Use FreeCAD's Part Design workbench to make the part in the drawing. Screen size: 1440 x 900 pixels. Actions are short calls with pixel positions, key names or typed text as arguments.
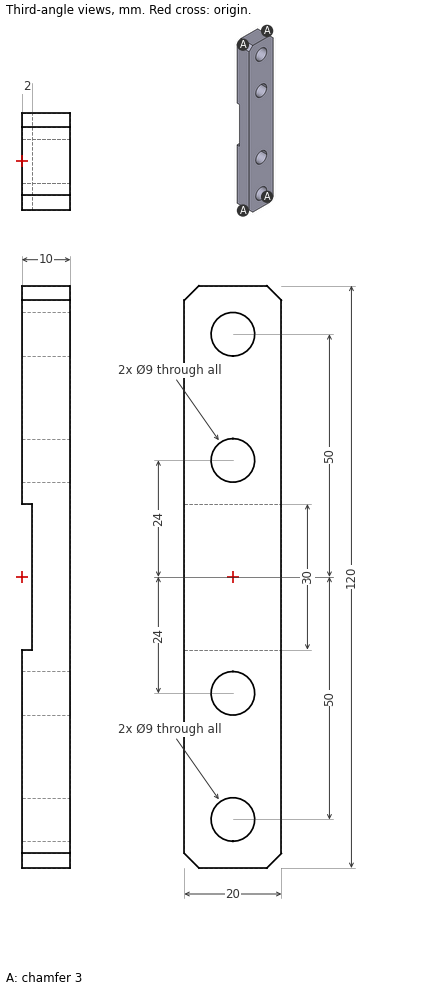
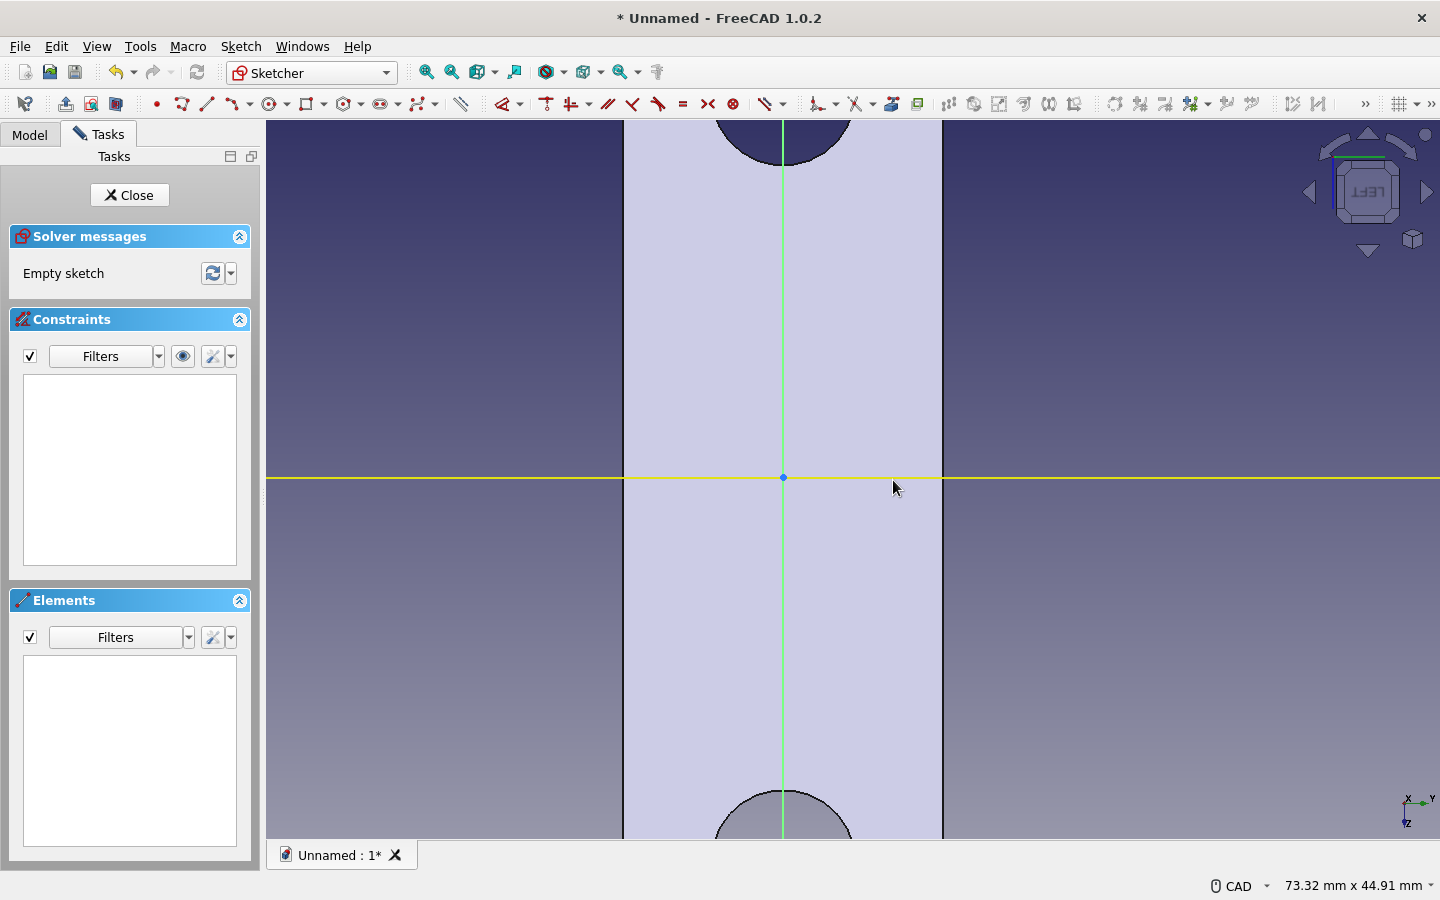
key(g)
key(v)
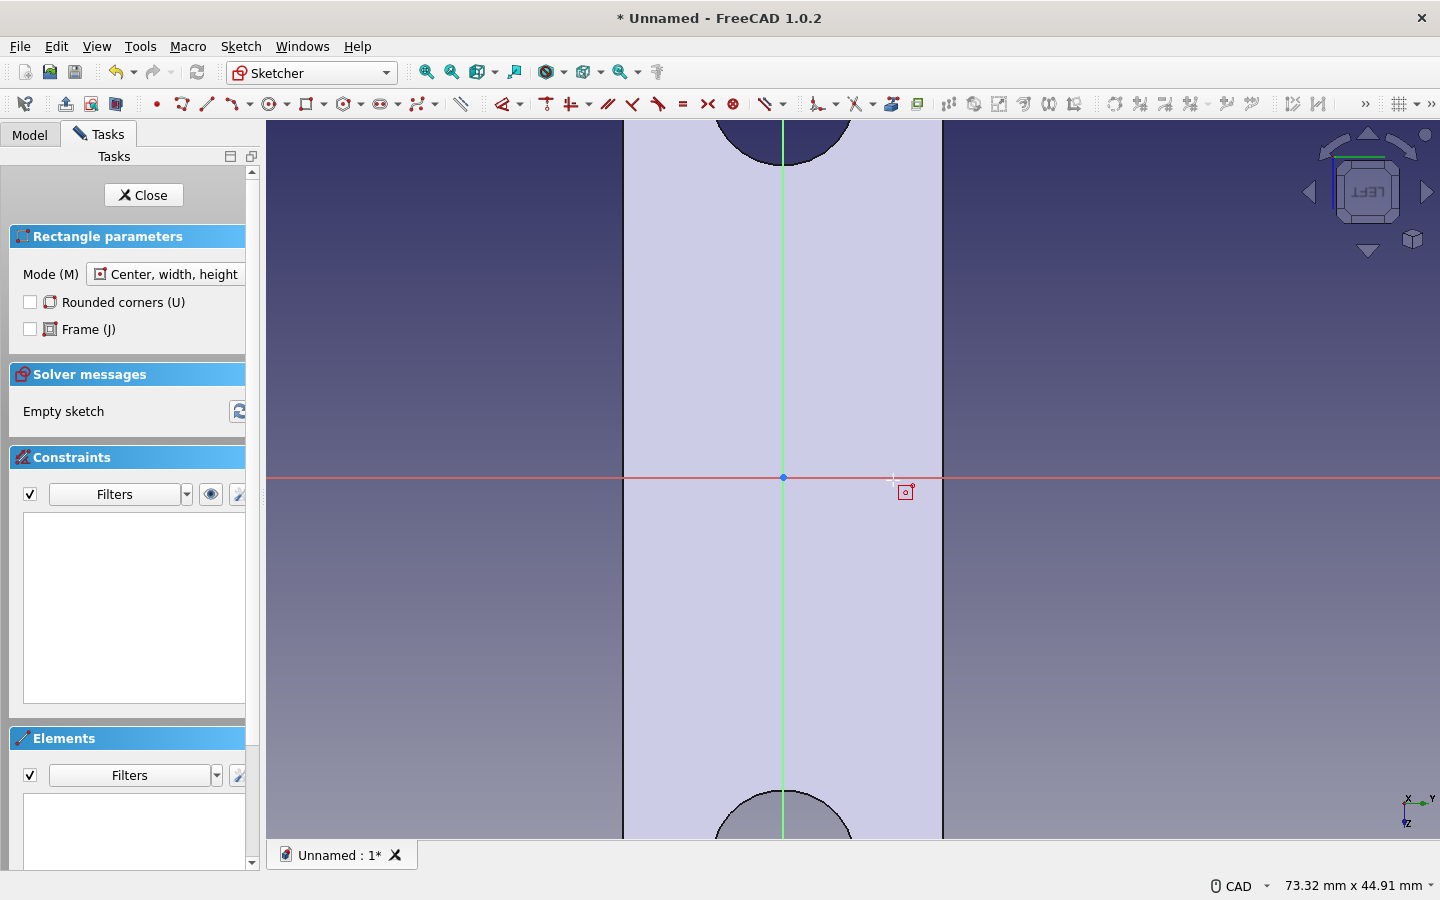
click(783, 478)
move(943, 238)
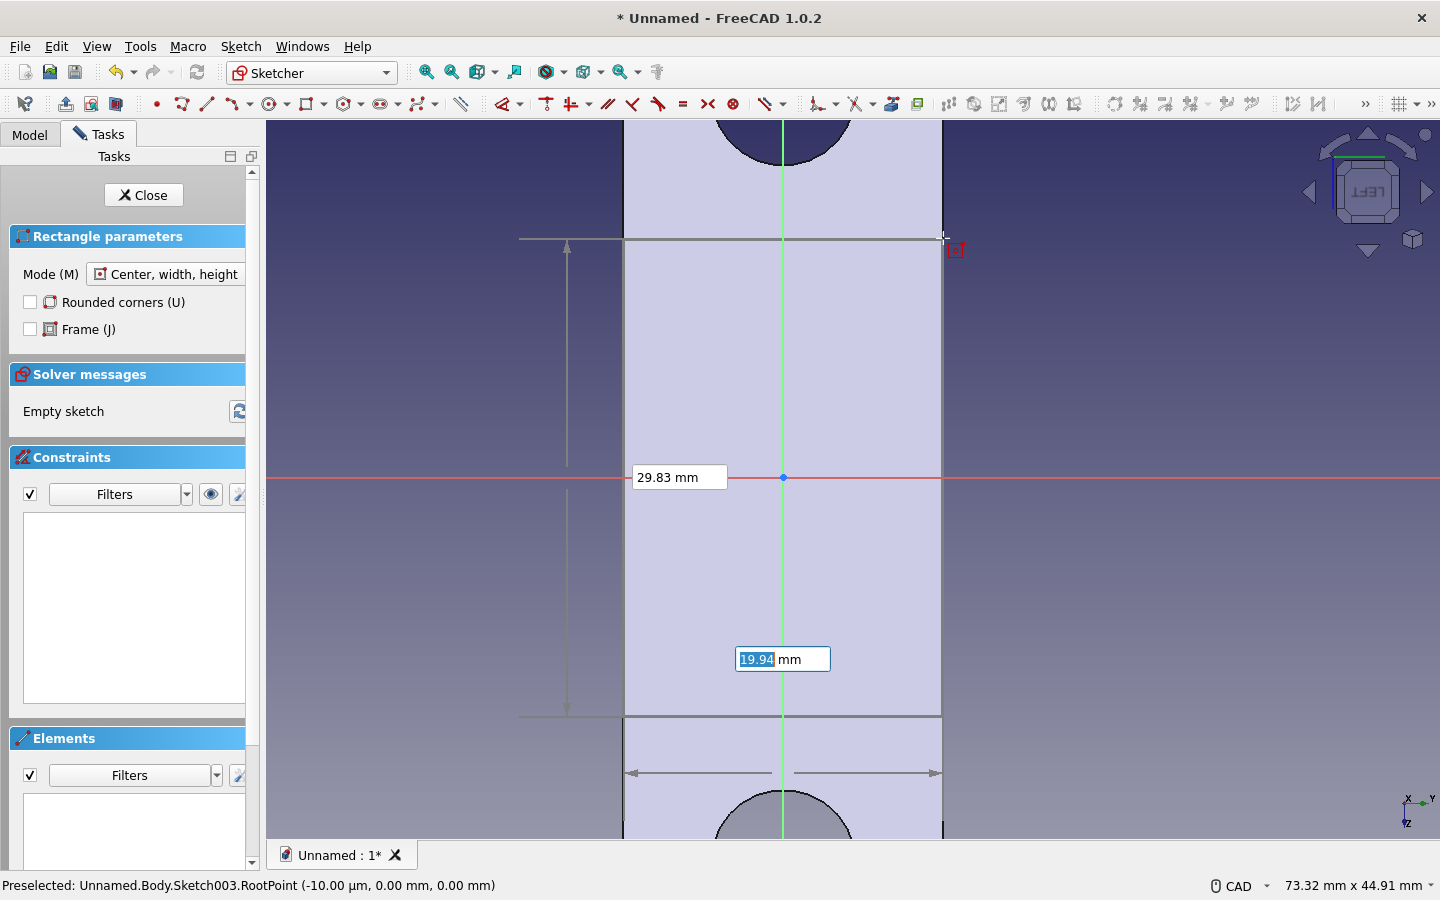
text(20)
key(Tab)
text(30)
key(Return)
key(Escape)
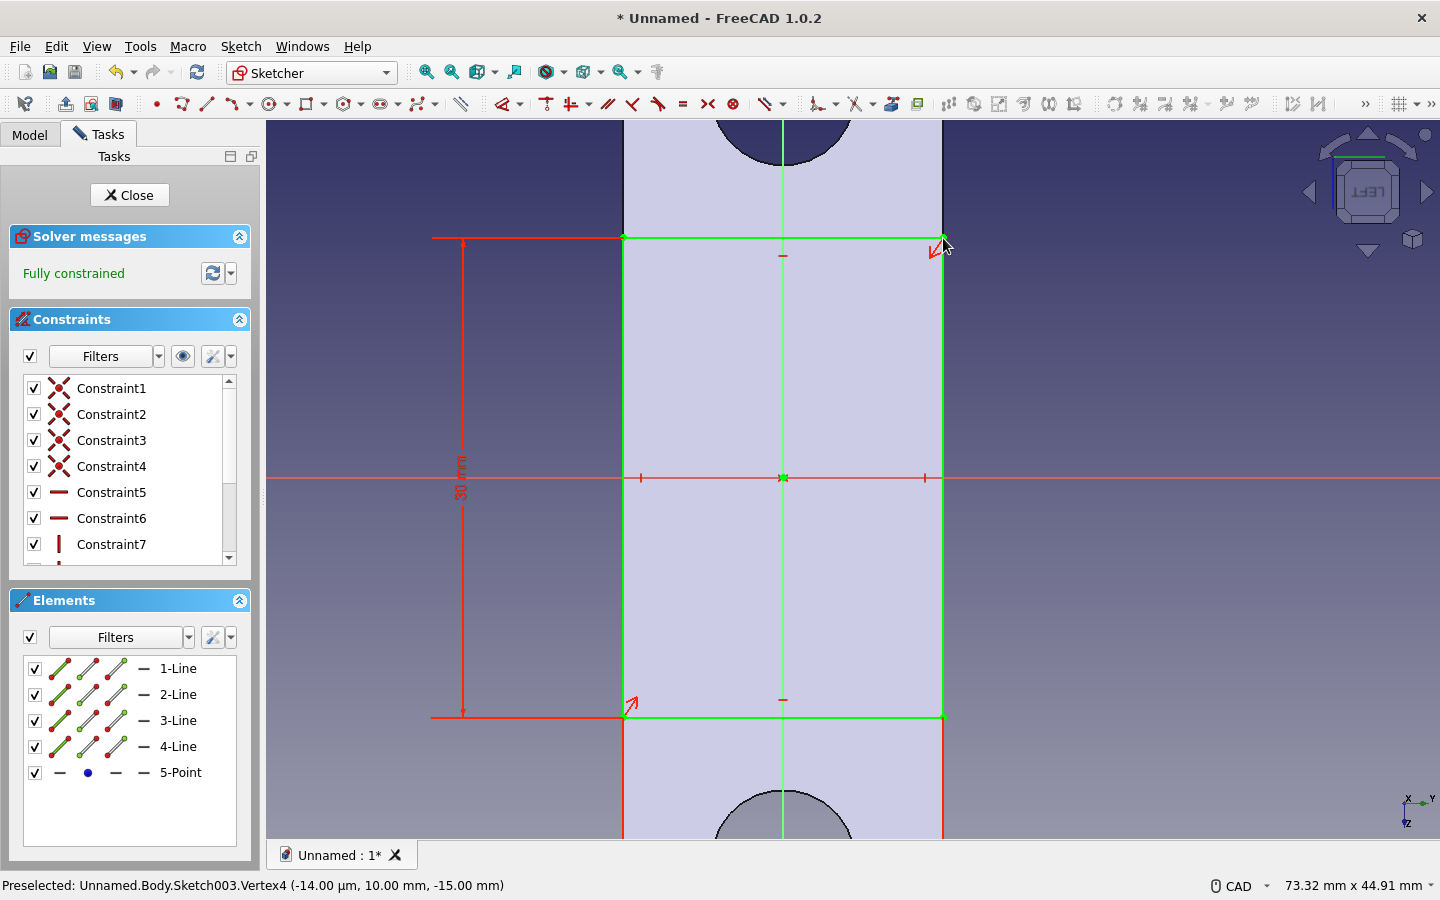
click(130, 195)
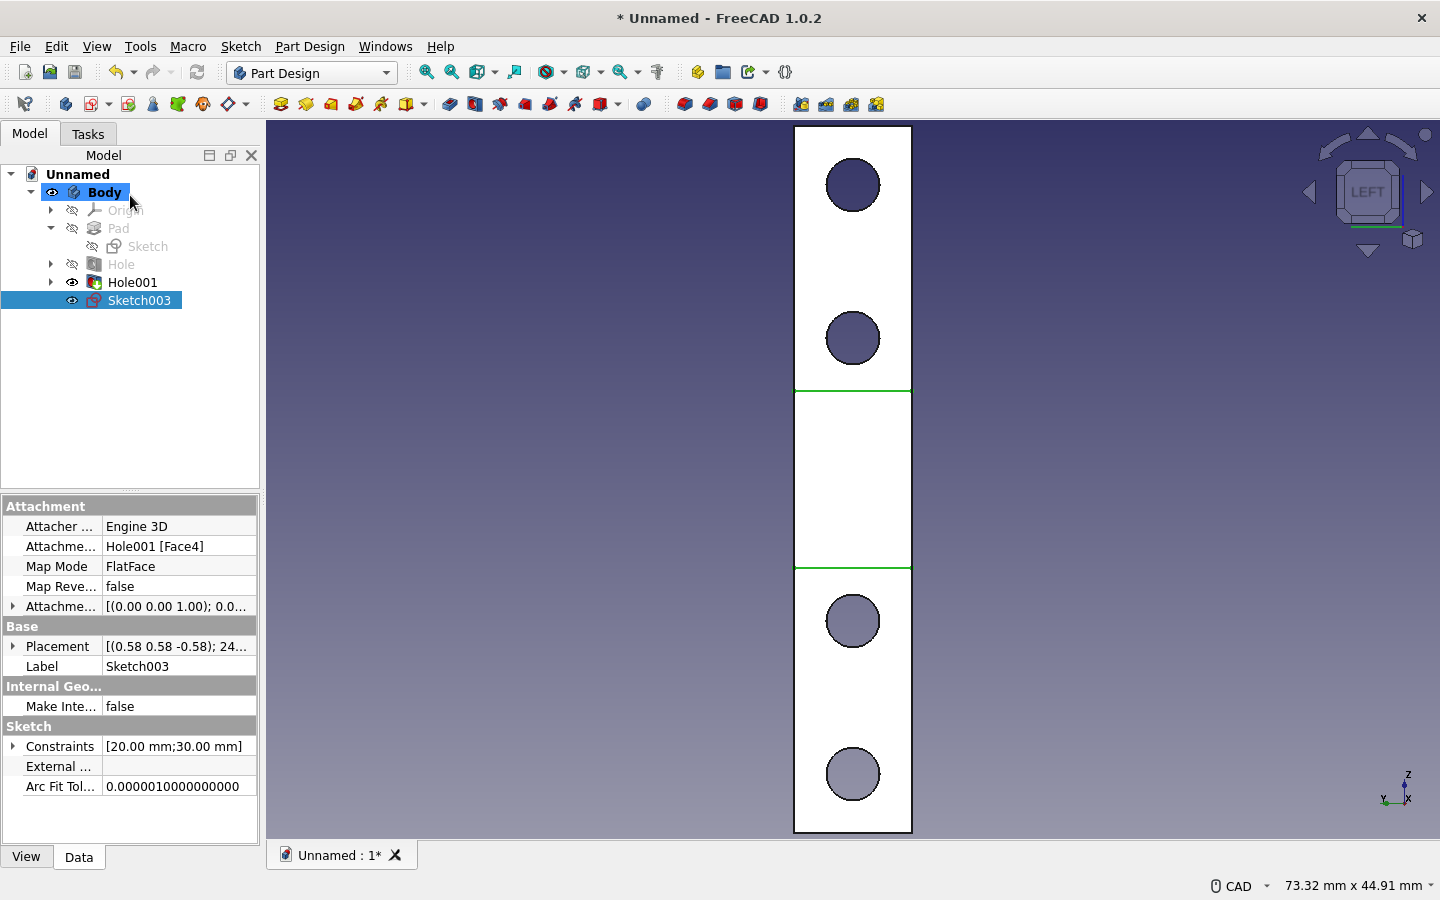
click(450, 104)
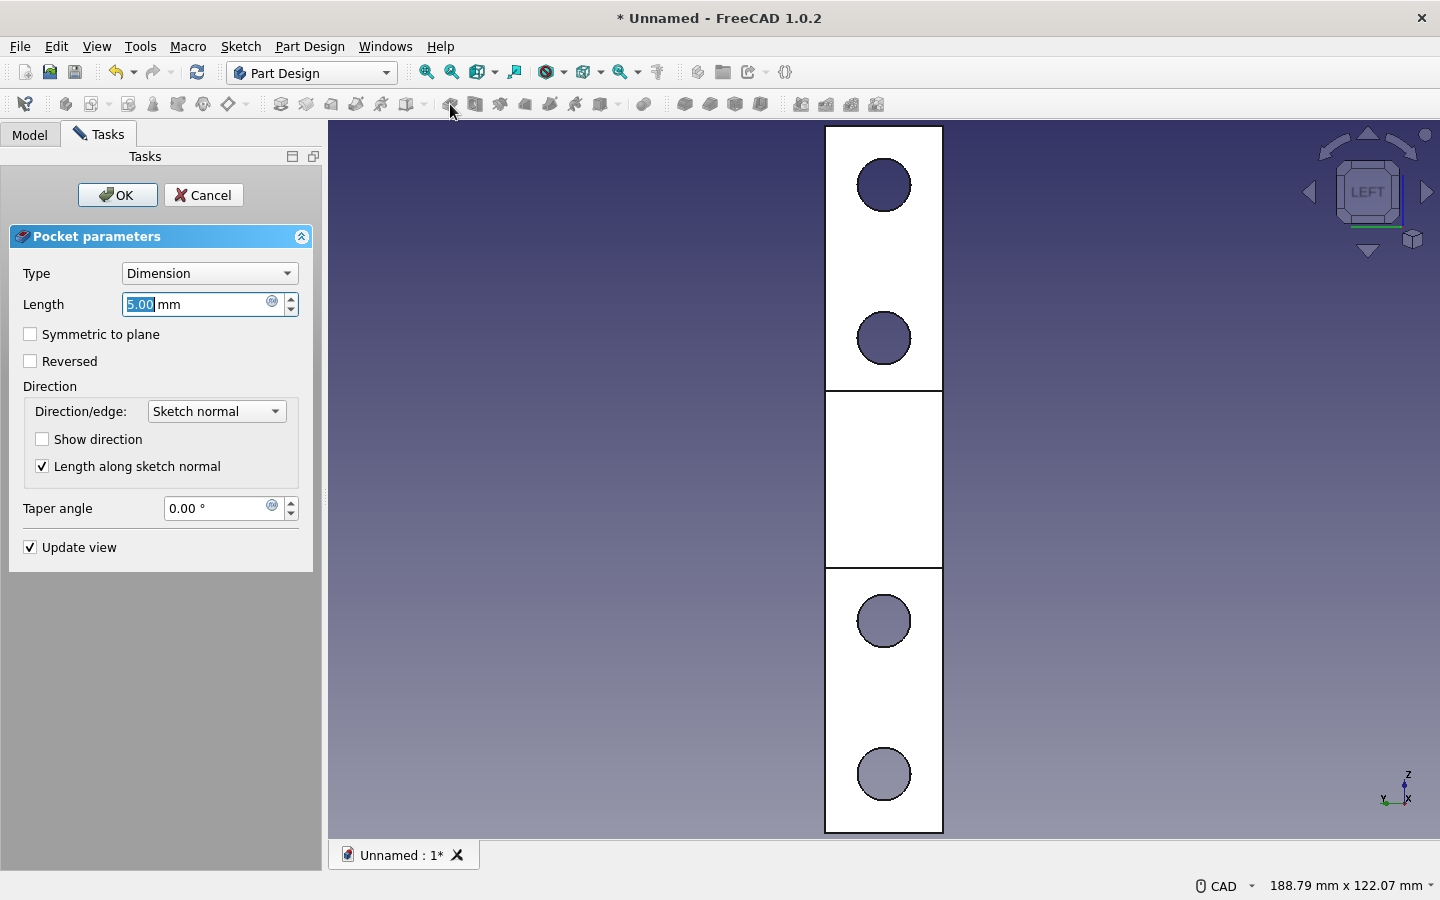
text(2)
key(Tab)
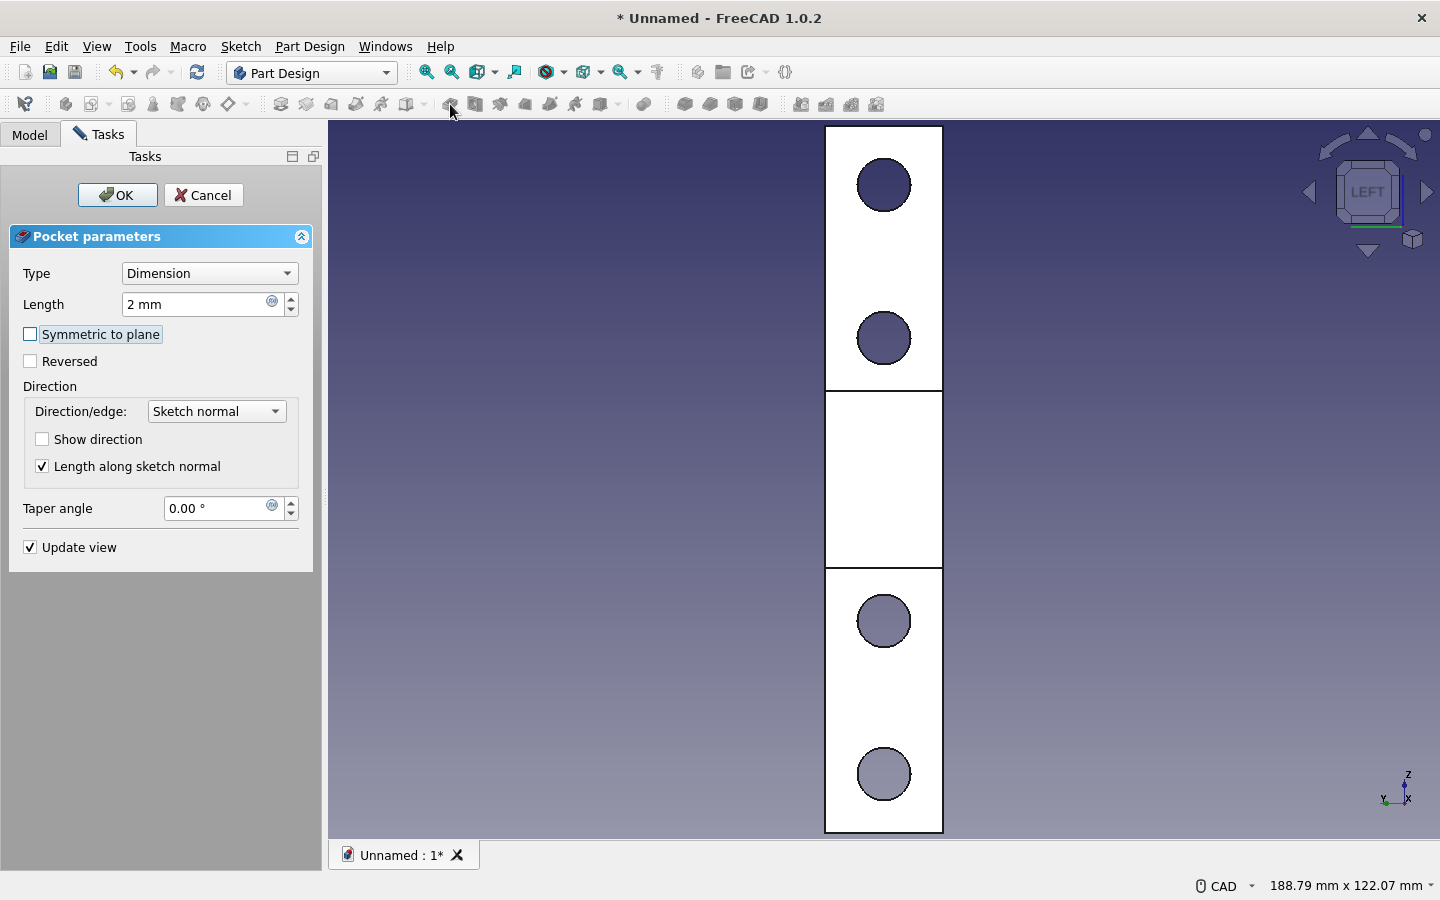
click(118, 195)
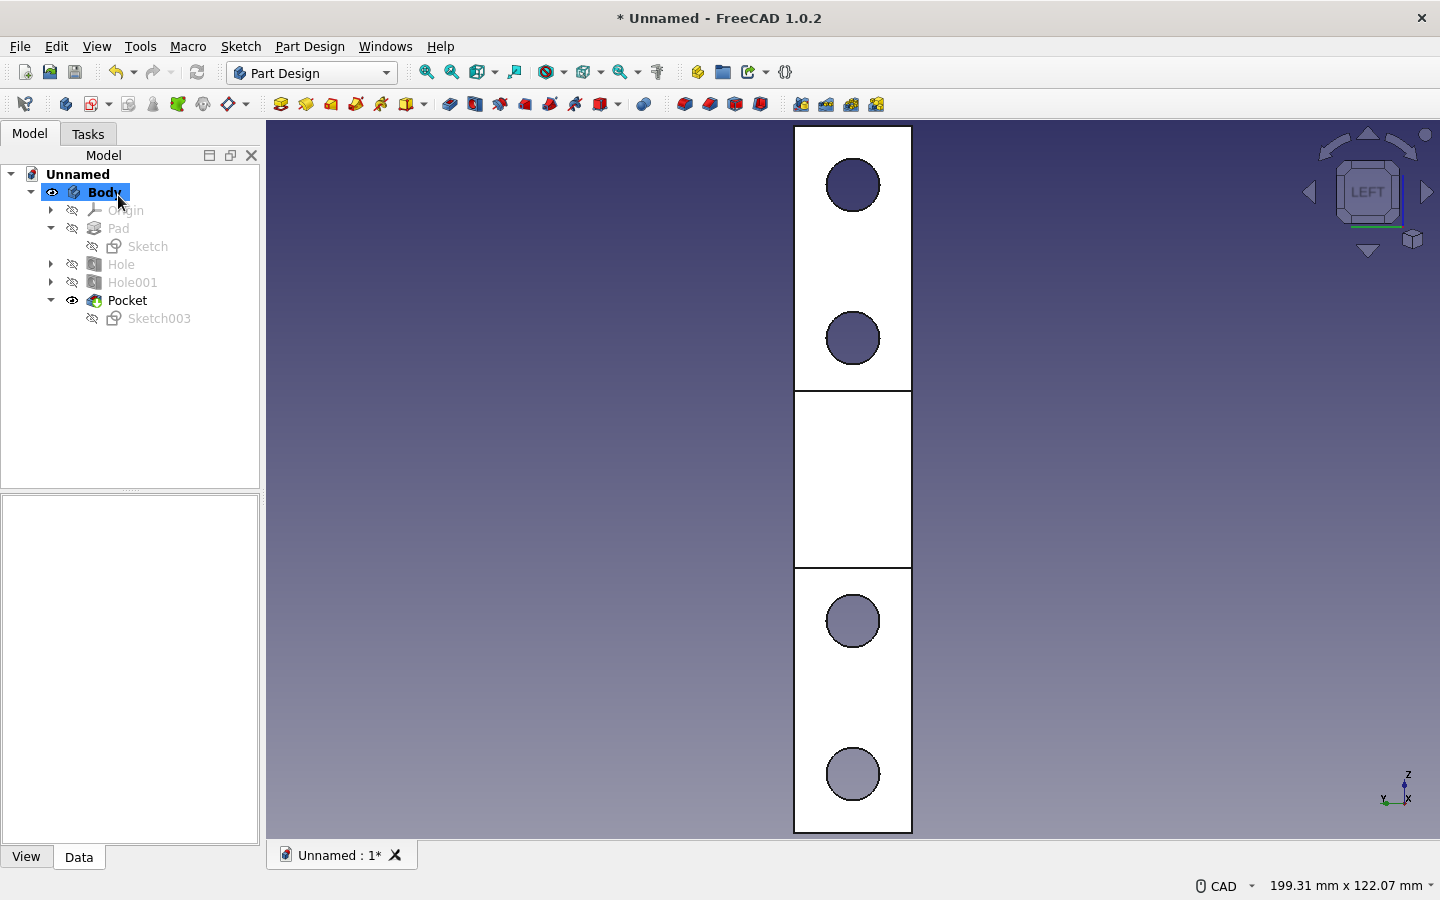
key(0)